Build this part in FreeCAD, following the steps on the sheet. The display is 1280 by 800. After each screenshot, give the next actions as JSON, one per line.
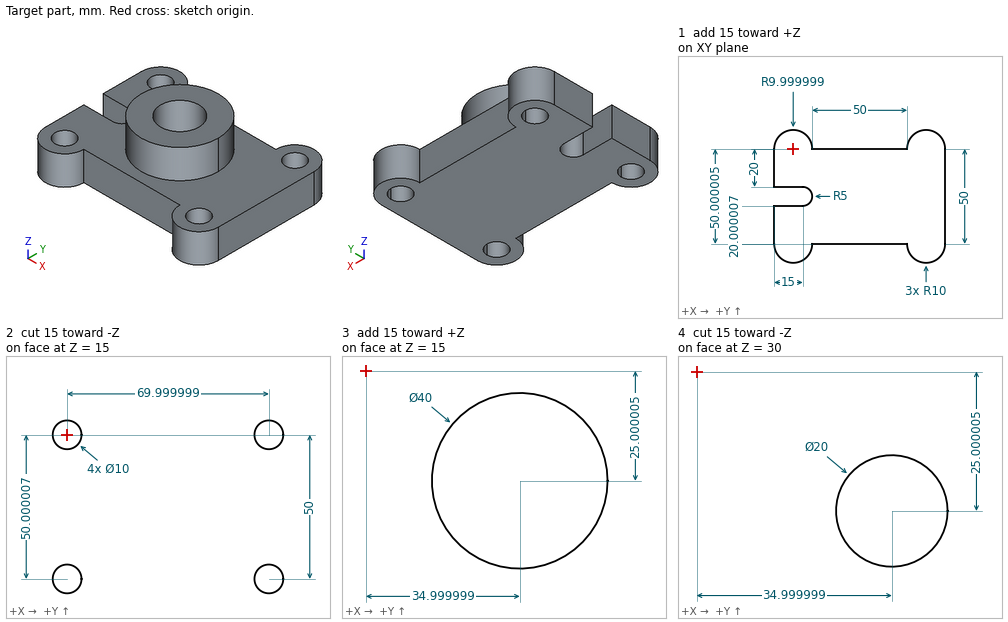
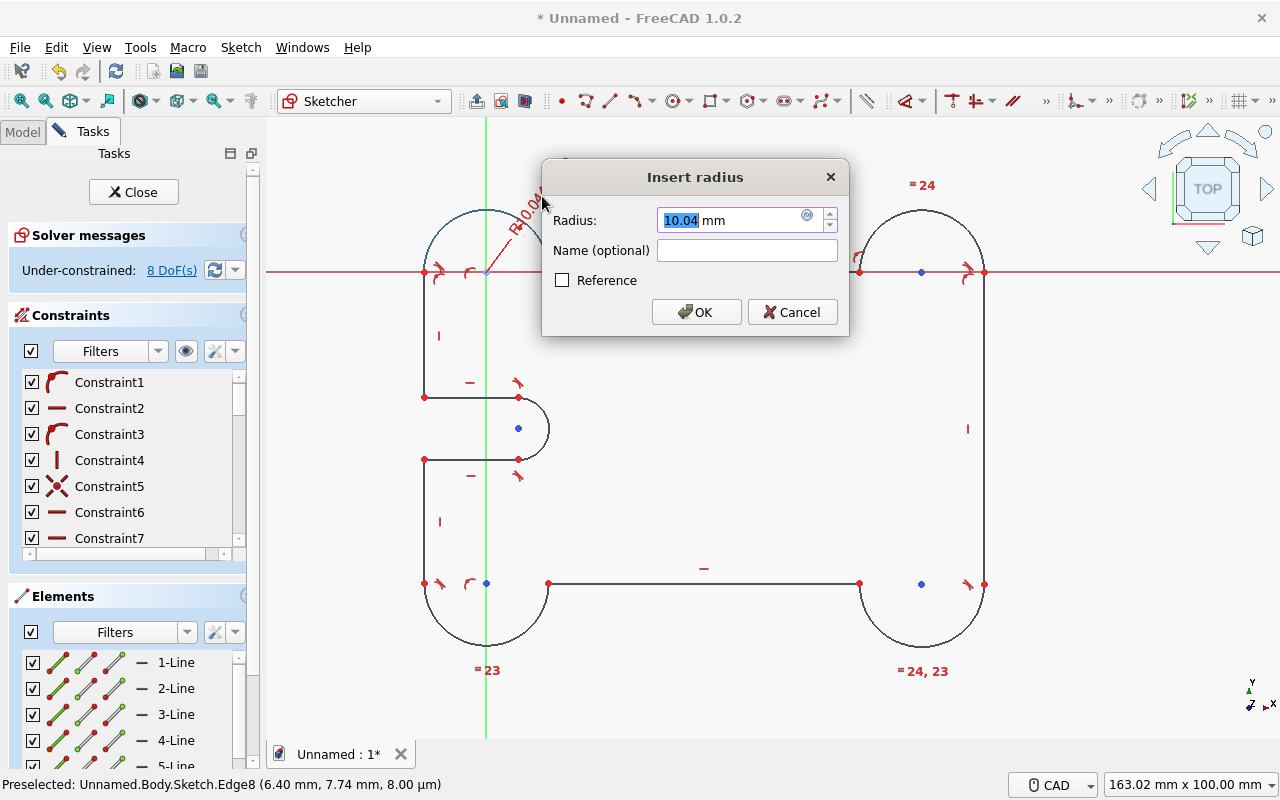
{"action": "type", "text": "9.999999"}
{"action": "key", "text": "Return"}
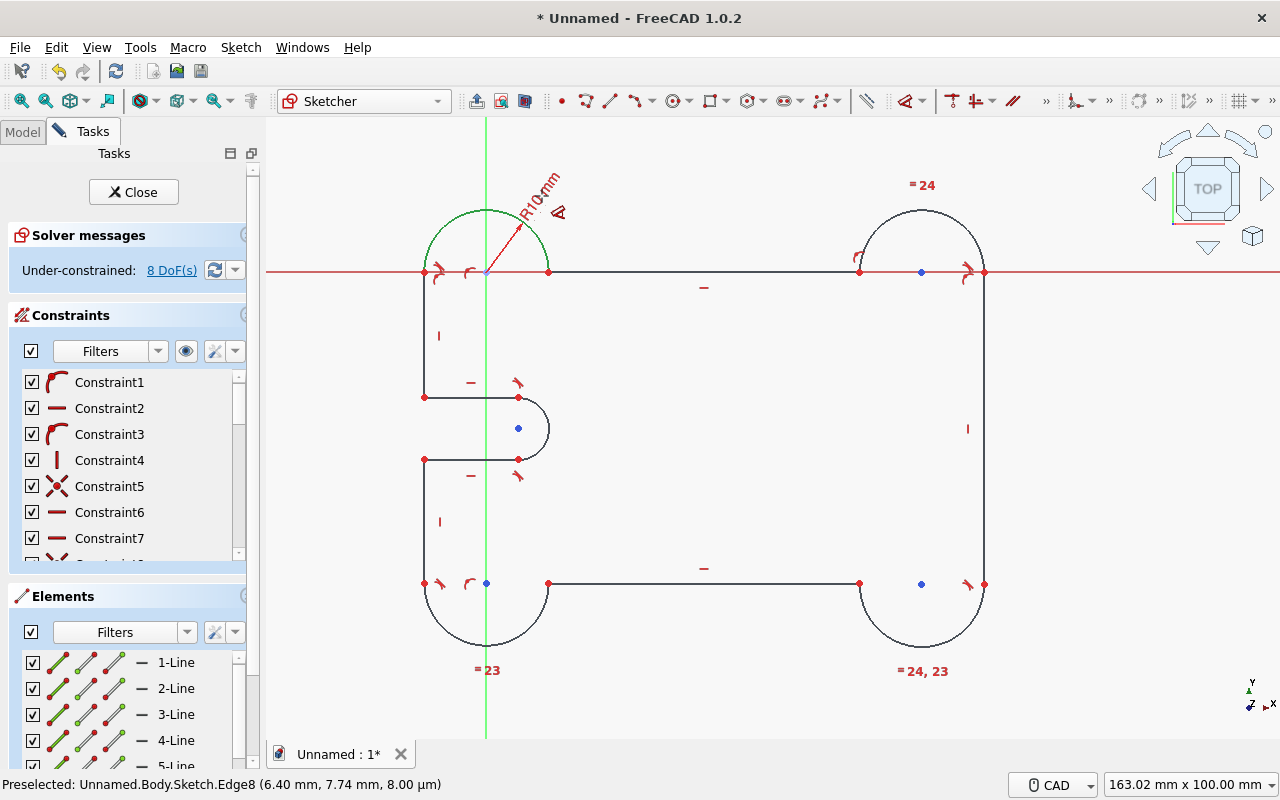
{"action": "scroll", "coordinate": [543, 447], "scroll_direction": "up", "scroll_amount": 2}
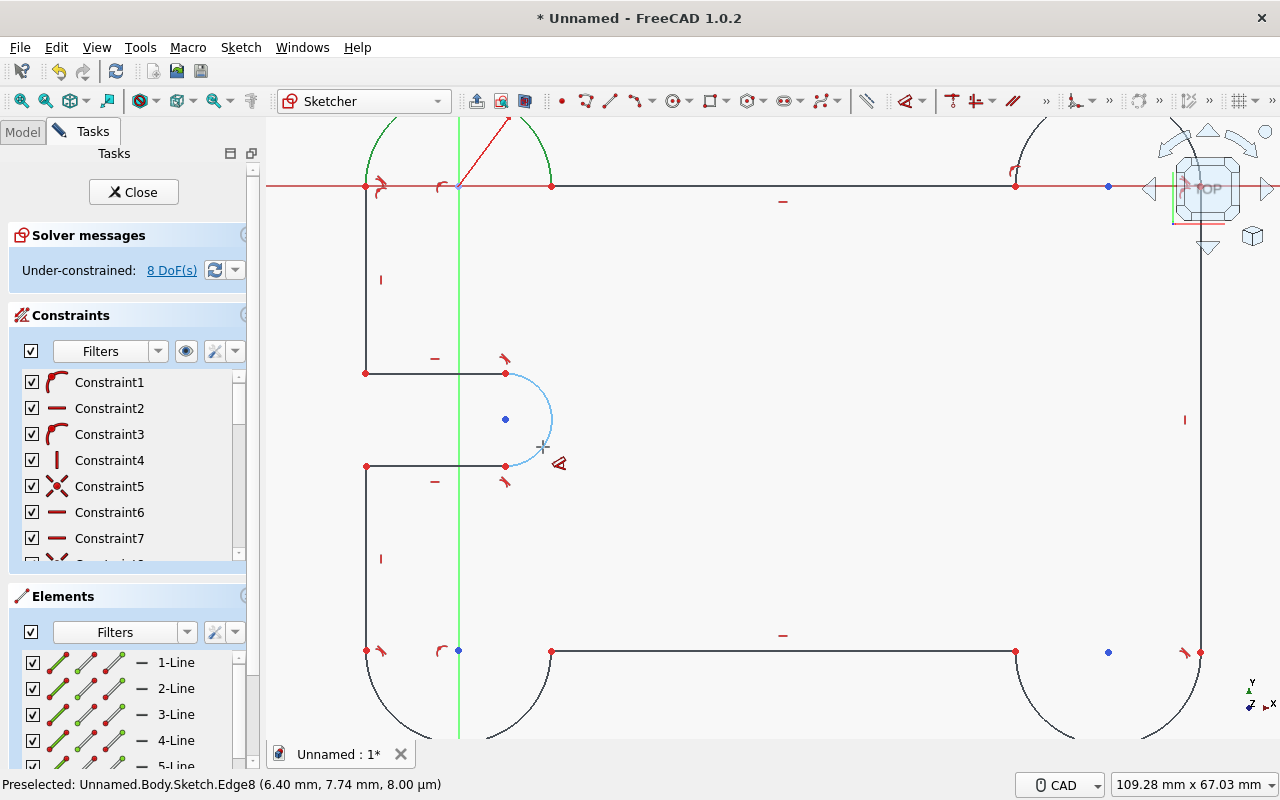
{"action": "left_click", "coordinate": [543, 447]}
{"action": "left_click", "coordinate": [569, 466]}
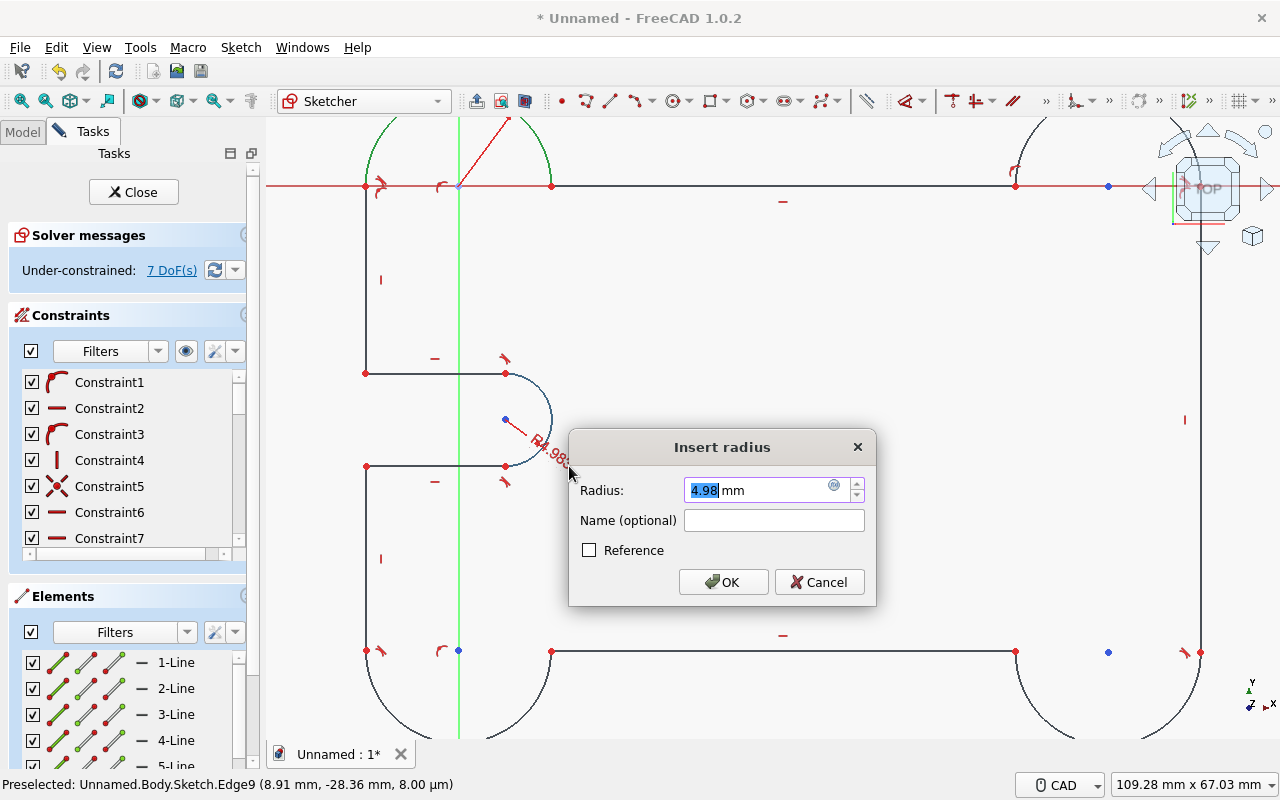
{"action": "type", "text": "5"}
{"action": "key", "text": "Return"}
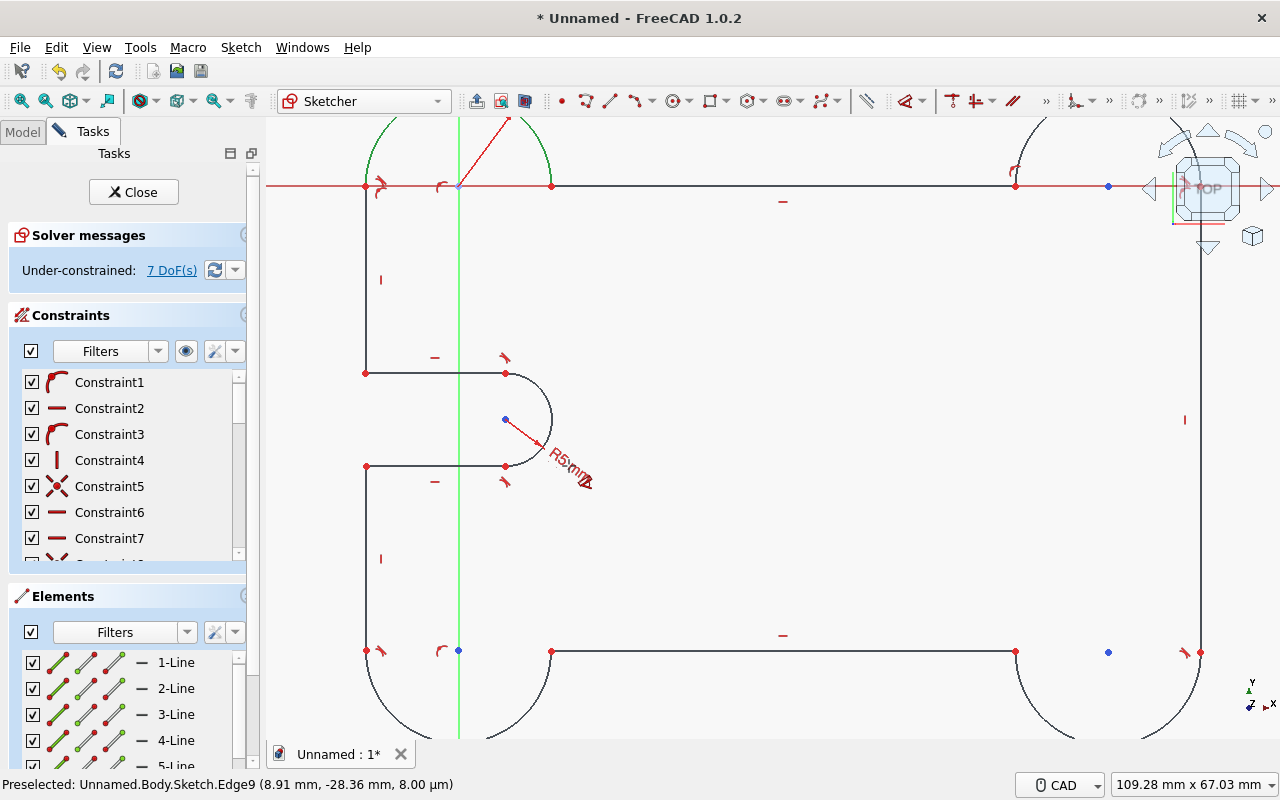
{"action": "left_click", "coordinate": [384, 705]}
{"action": "left_click", "coordinate": [335, 667]}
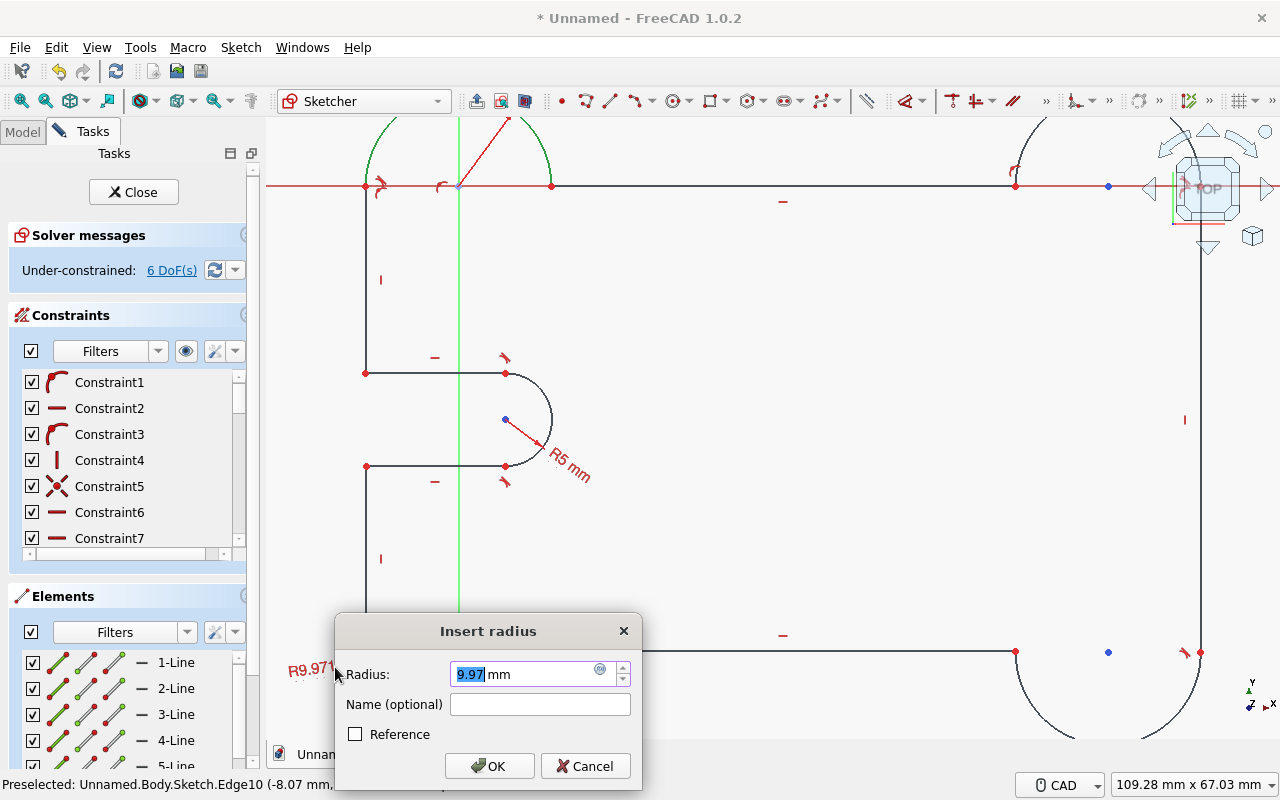
{"action": "type", "text": "10"}
{"action": "key", "text": "Return"}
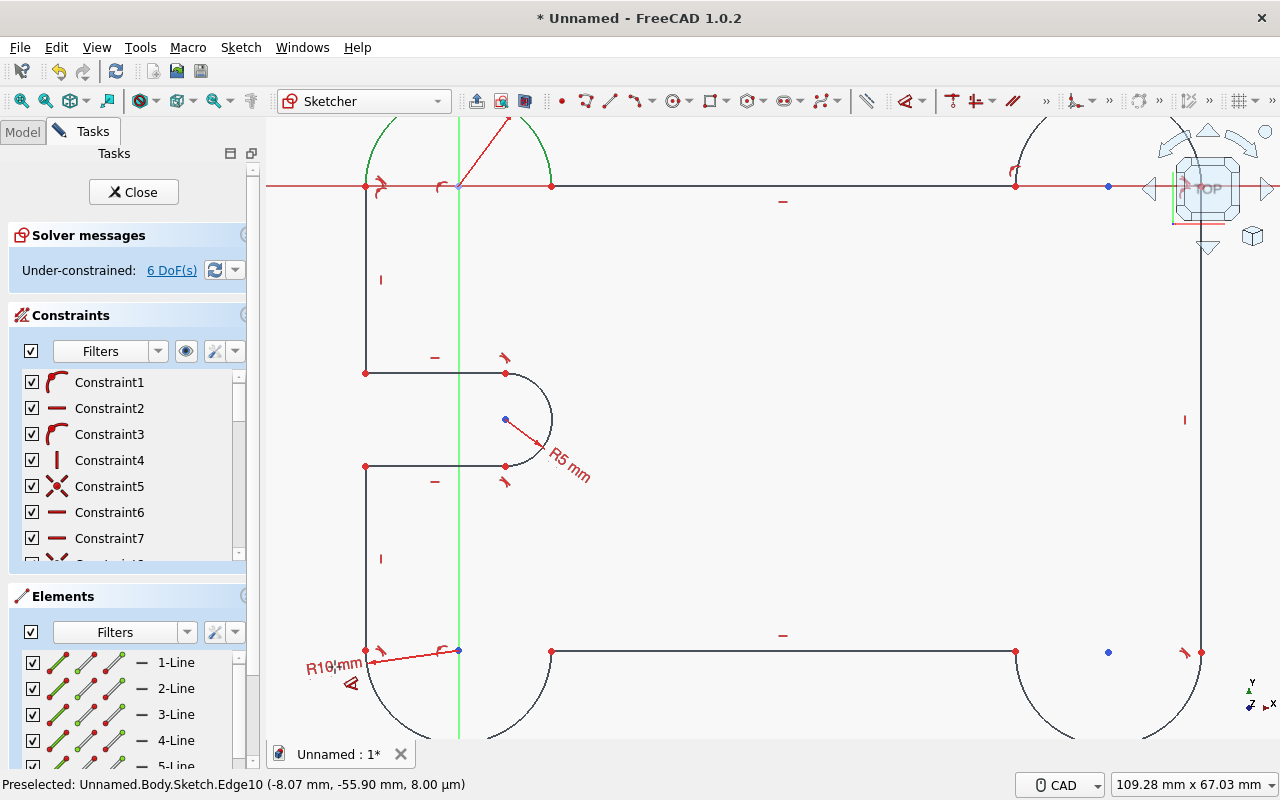
{"action": "left_click", "coordinate": [876, 186]}
{"action": "left_click", "coordinate": [784, 152]}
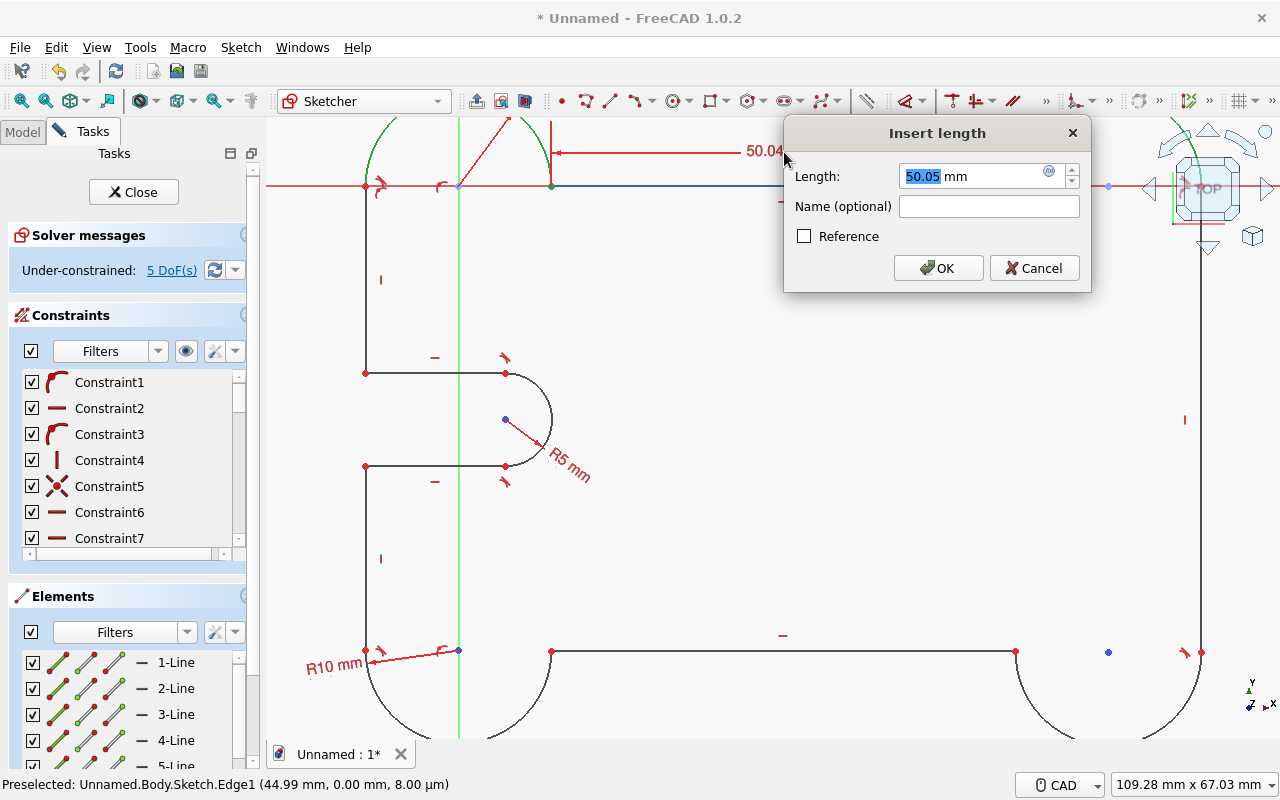
{"action": "type", "text": "50"}
{"action": "key", "text": "Return"}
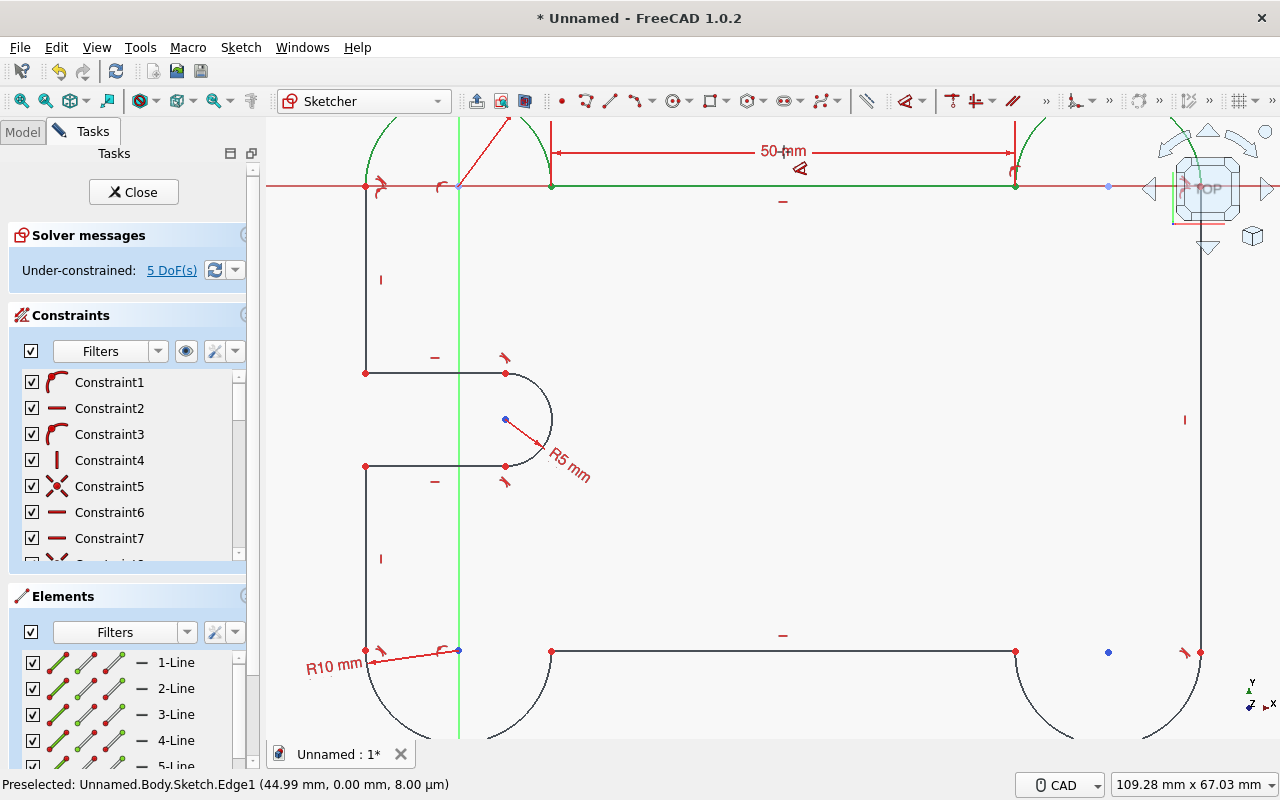
{"action": "left_click", "coordinate": [366, 242]}
{"action": "left_click", "coordinate": [332, 280]}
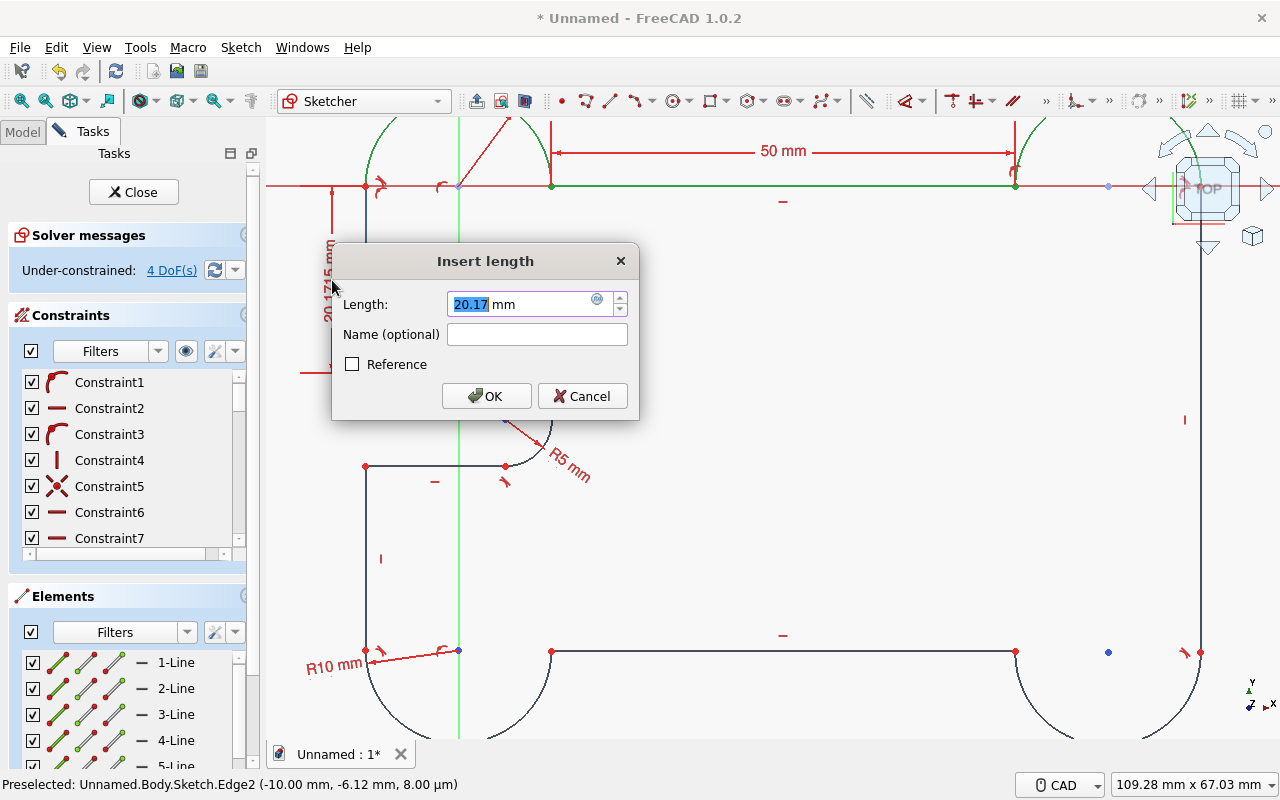
{"action": "type", "text": "20"}
{"action": "key", "text": "Return"}